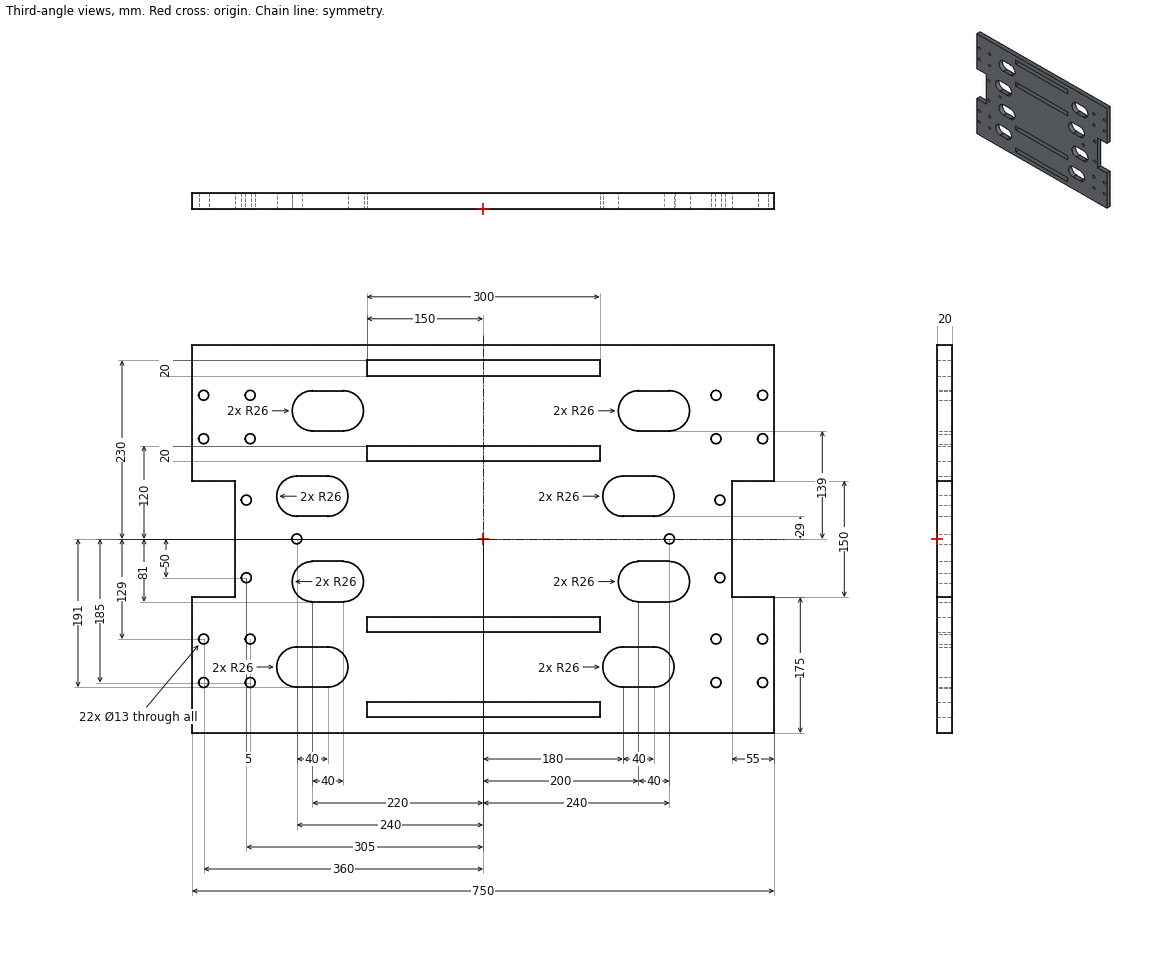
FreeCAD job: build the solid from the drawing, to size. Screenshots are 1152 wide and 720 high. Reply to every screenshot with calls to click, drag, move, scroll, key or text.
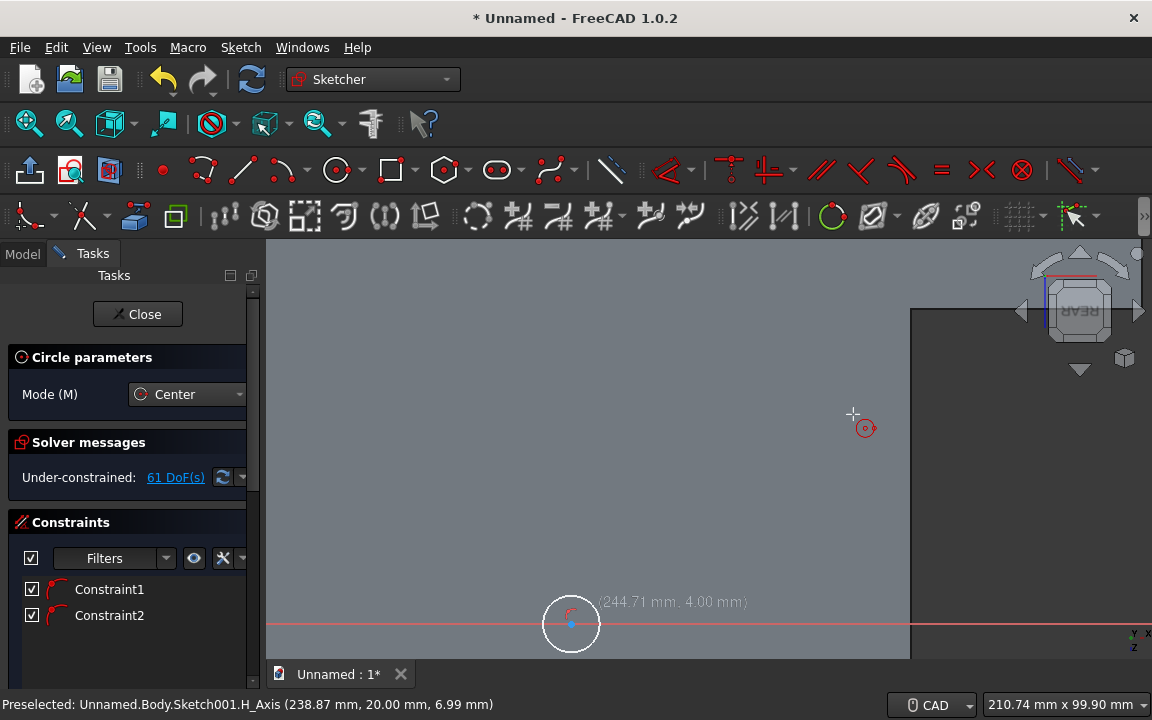
scroll(853, 414, down, 9)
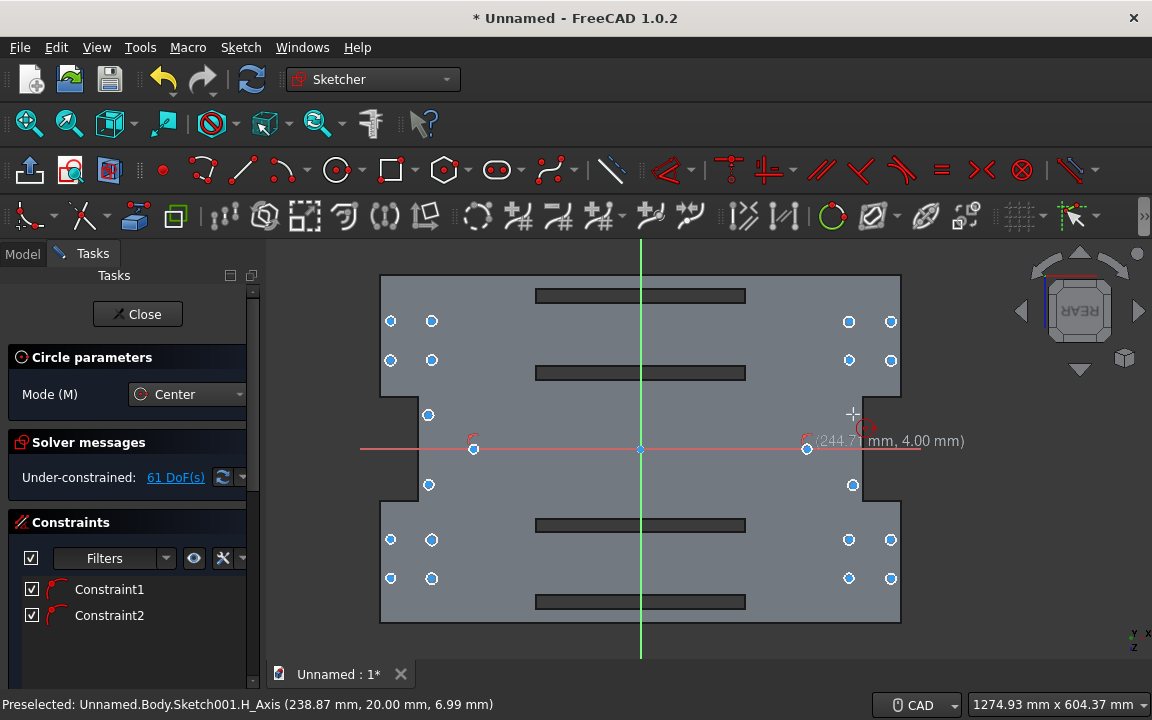
click(853, 414)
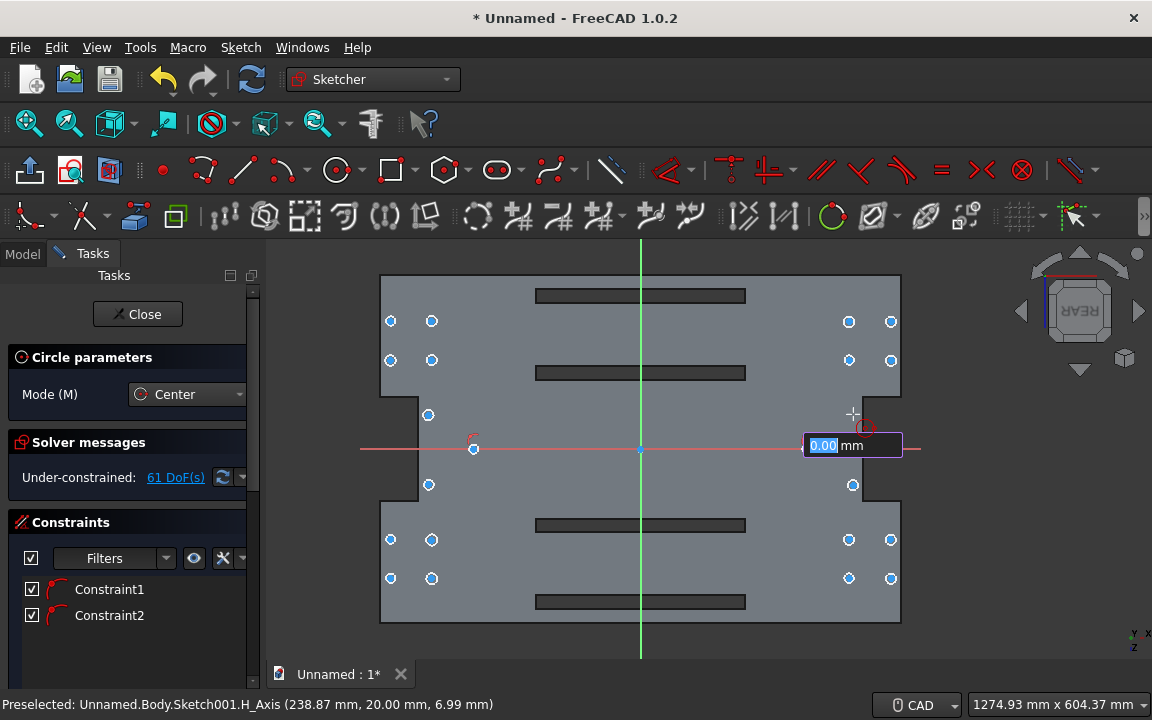
scroll(856, 411, up, 7)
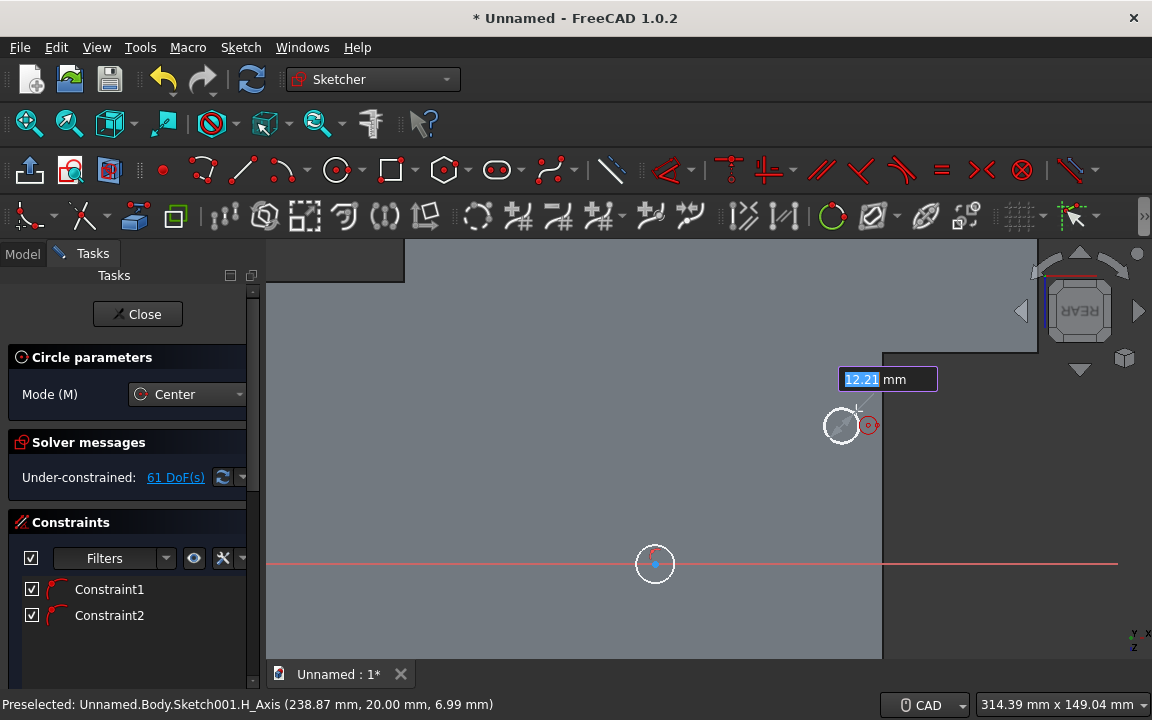
click(853, 410)
key(Escape)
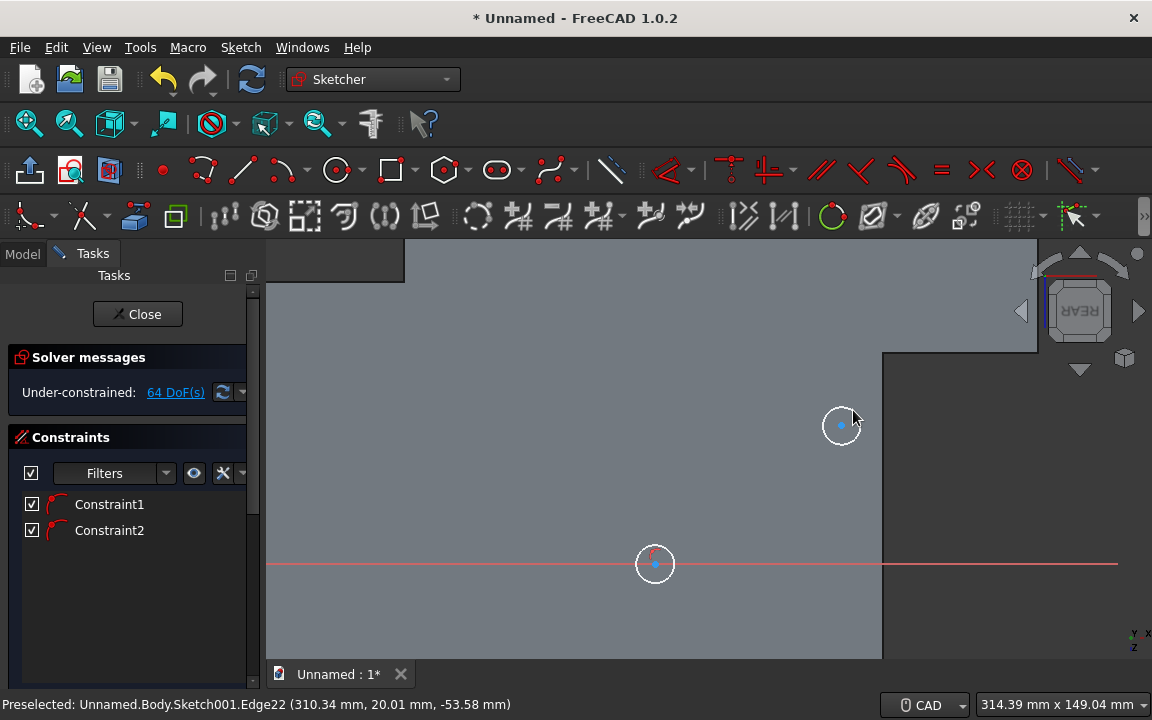
scroll(856, 411, down, 7)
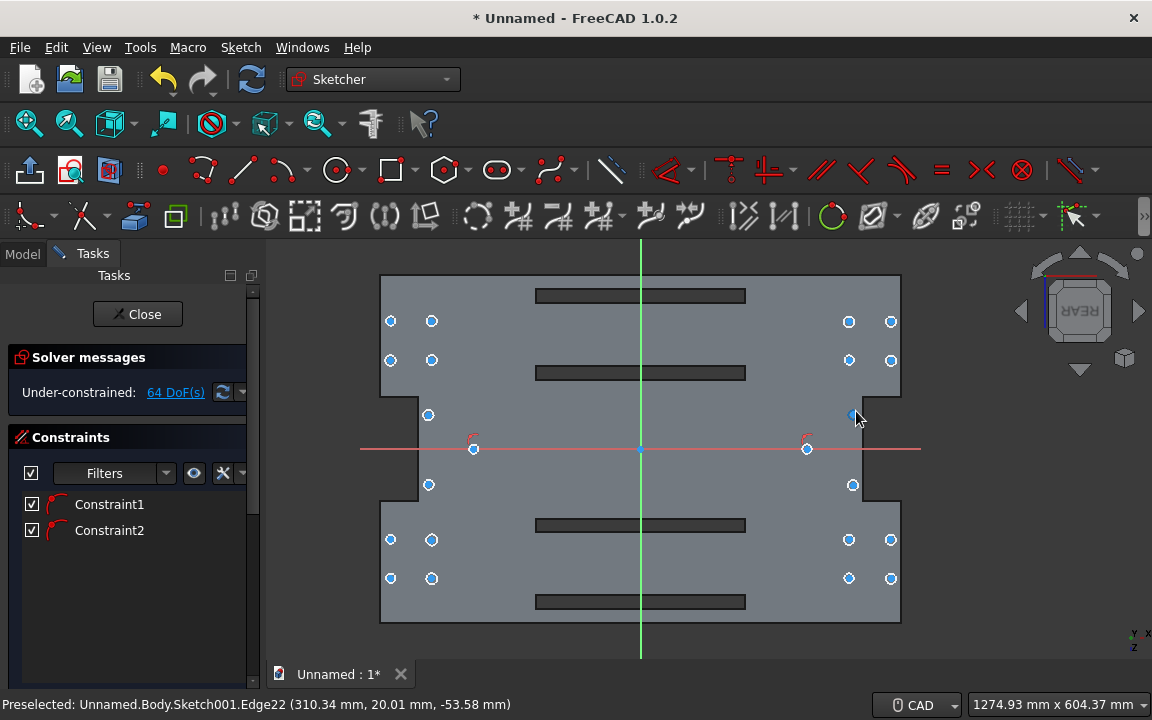
scroll(394, 357, up, 5)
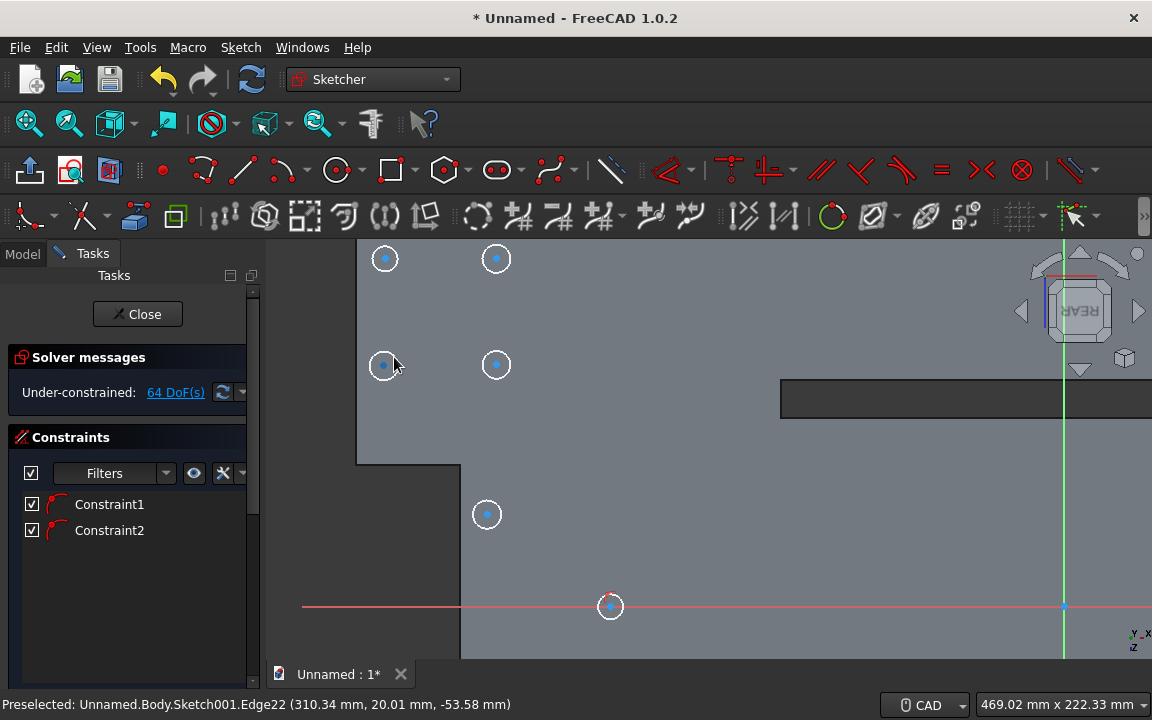
click(394, 356)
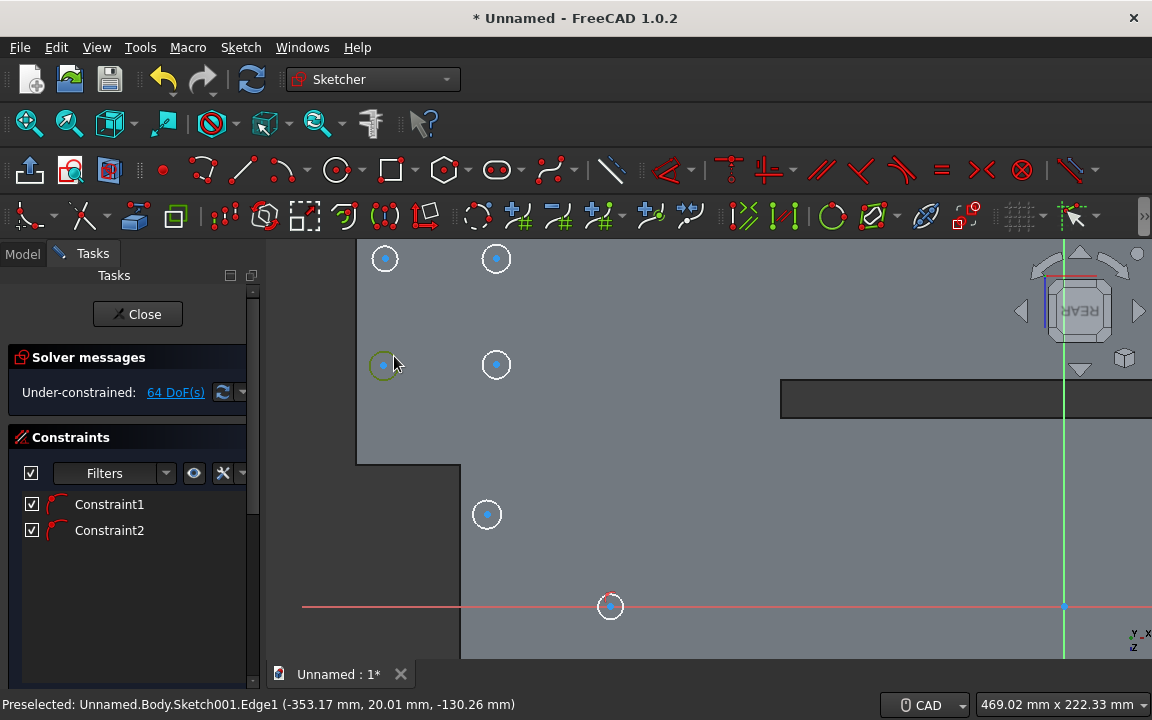
click(497, 505)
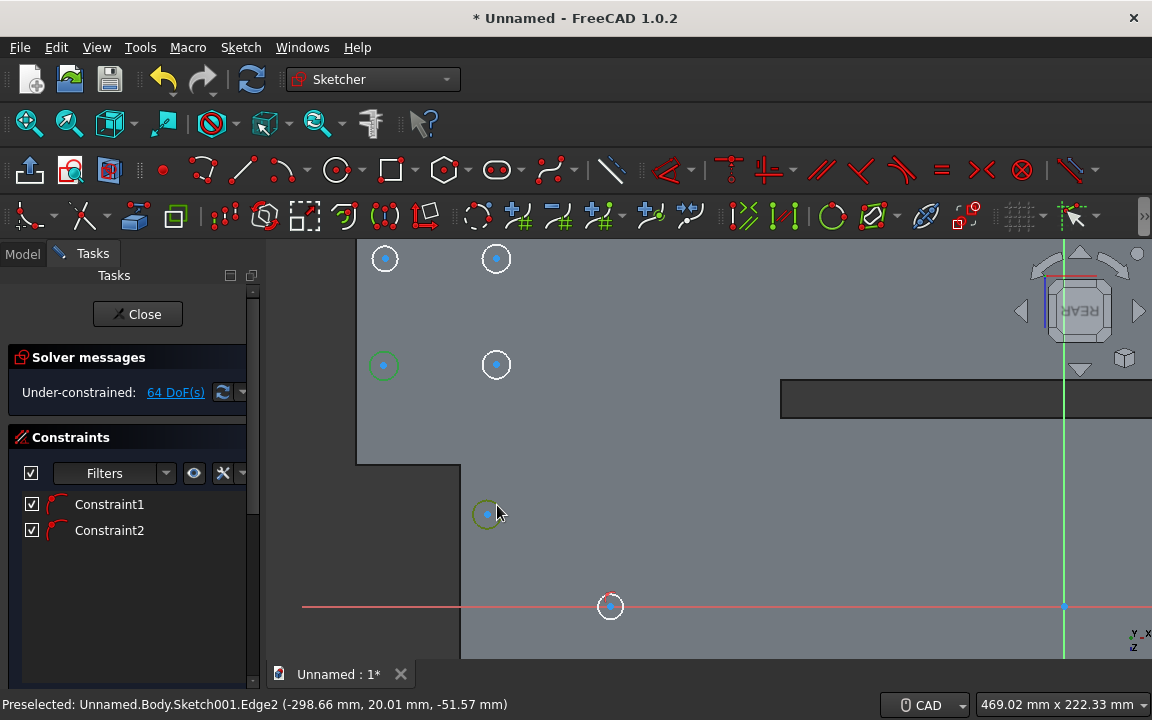
click(598, 606)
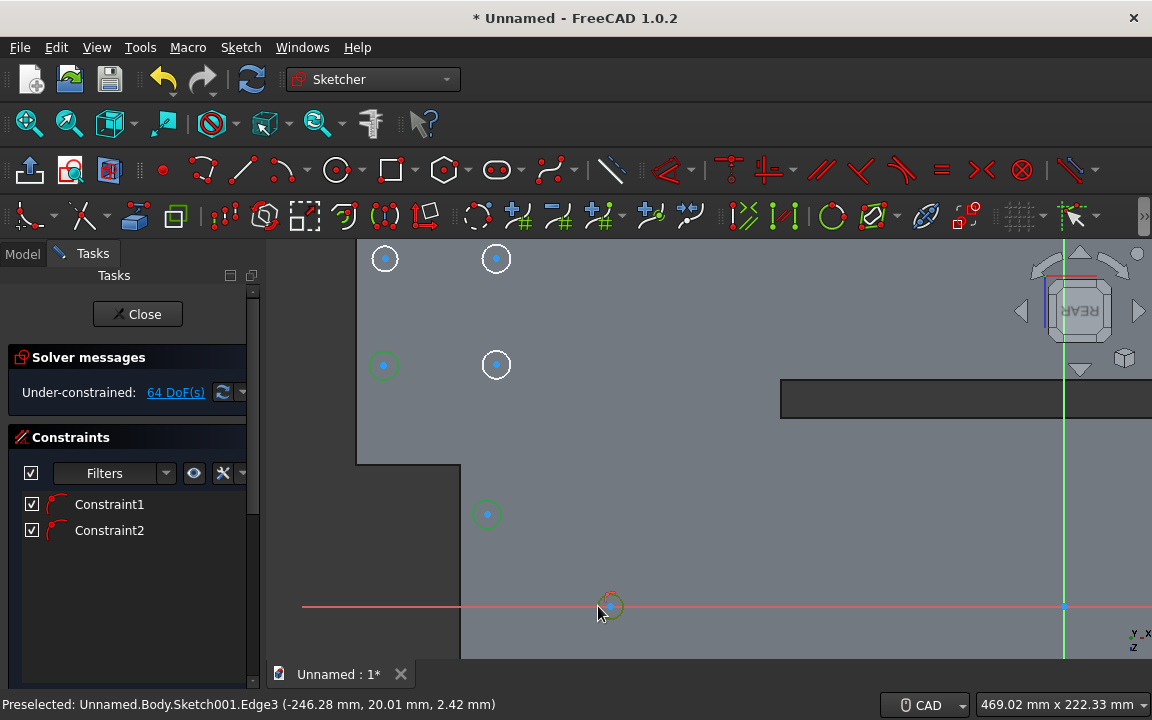
click(506, 355)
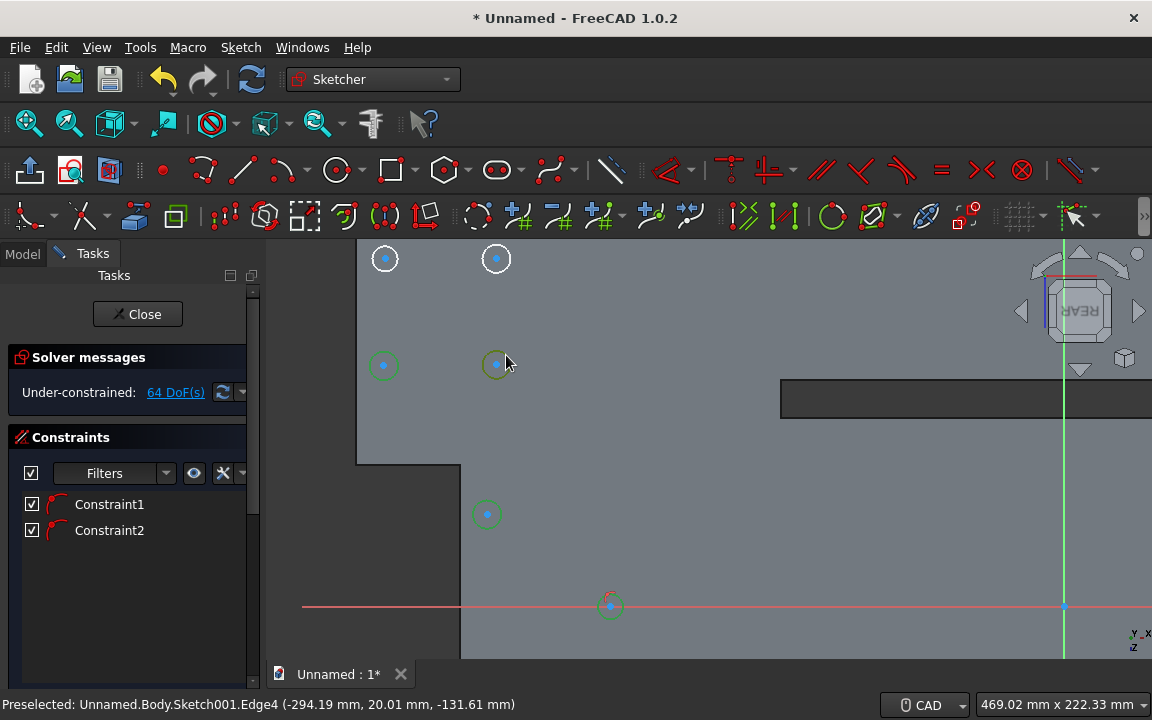
click(487, 269)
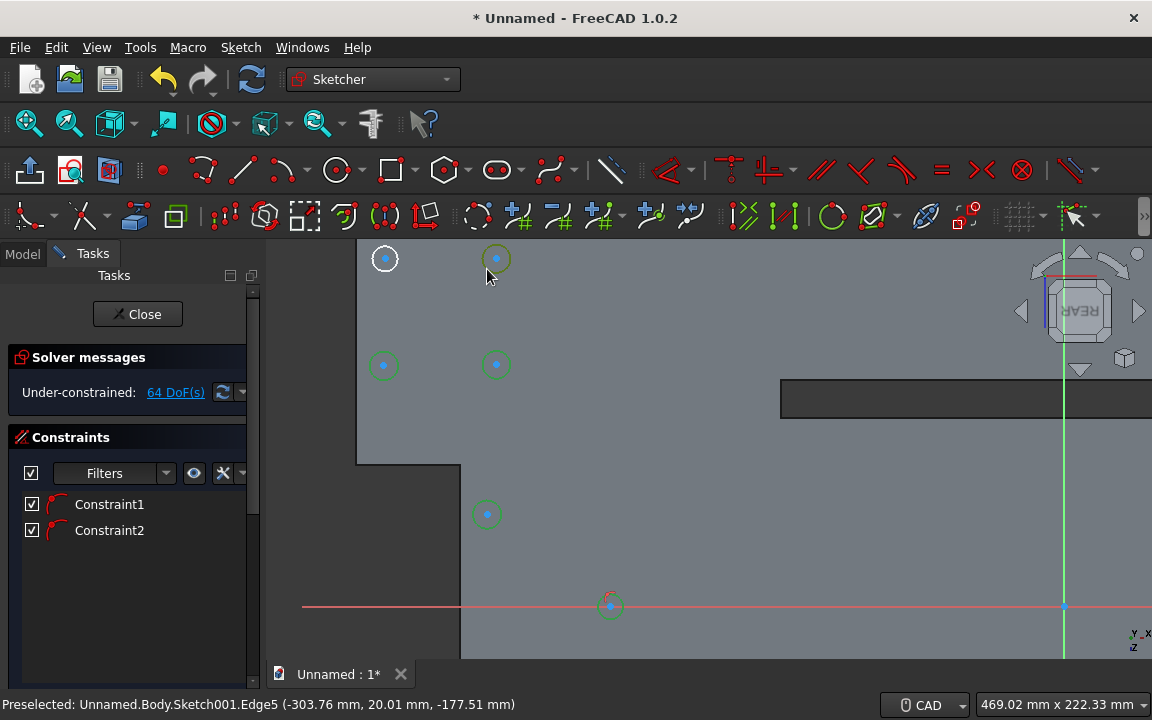
click(376, 268)